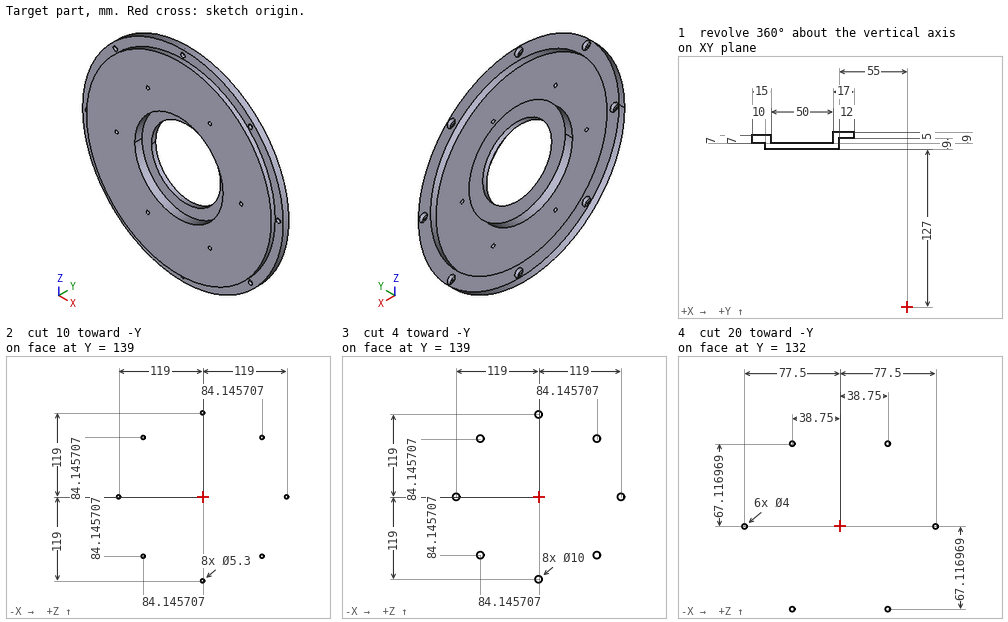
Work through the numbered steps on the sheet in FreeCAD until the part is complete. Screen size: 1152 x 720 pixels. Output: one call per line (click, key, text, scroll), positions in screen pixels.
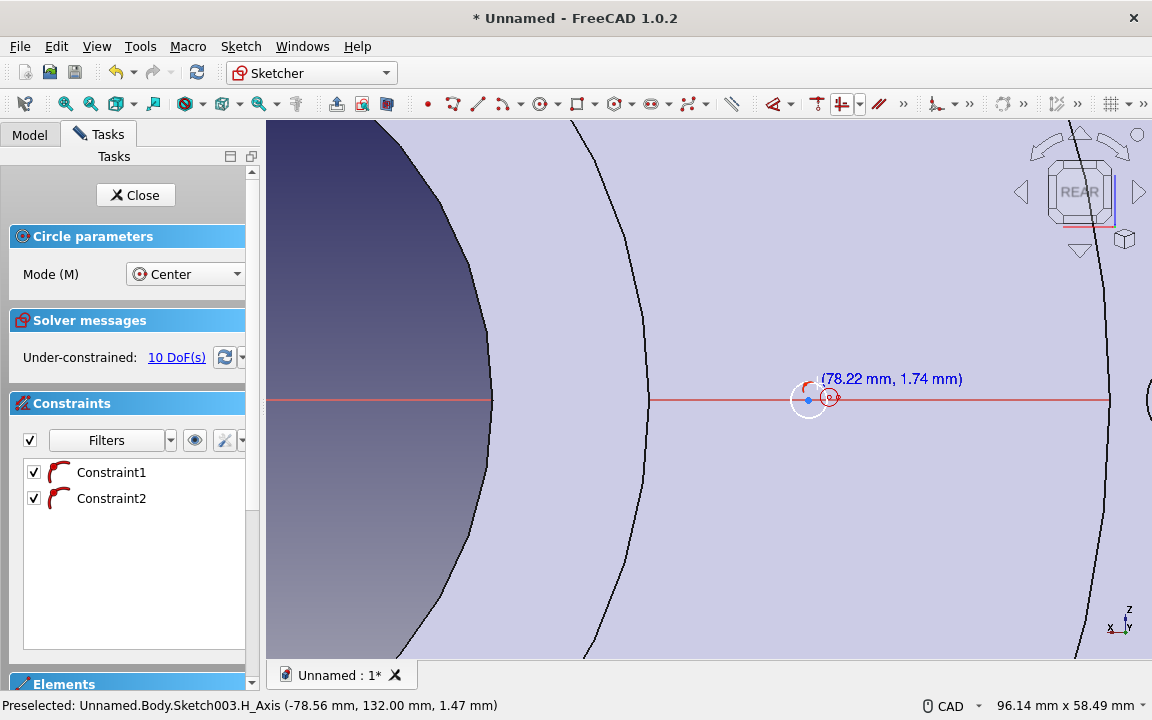
scroll(819, 386, down, 7)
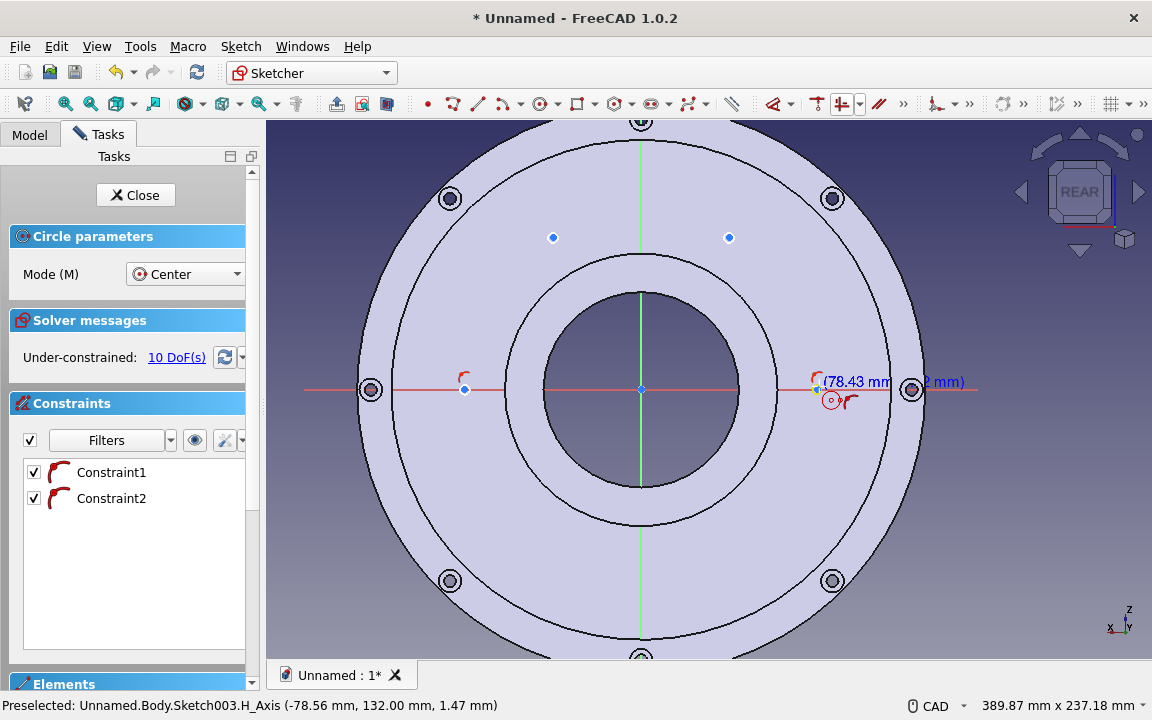
scroll(729, 542, up, 9)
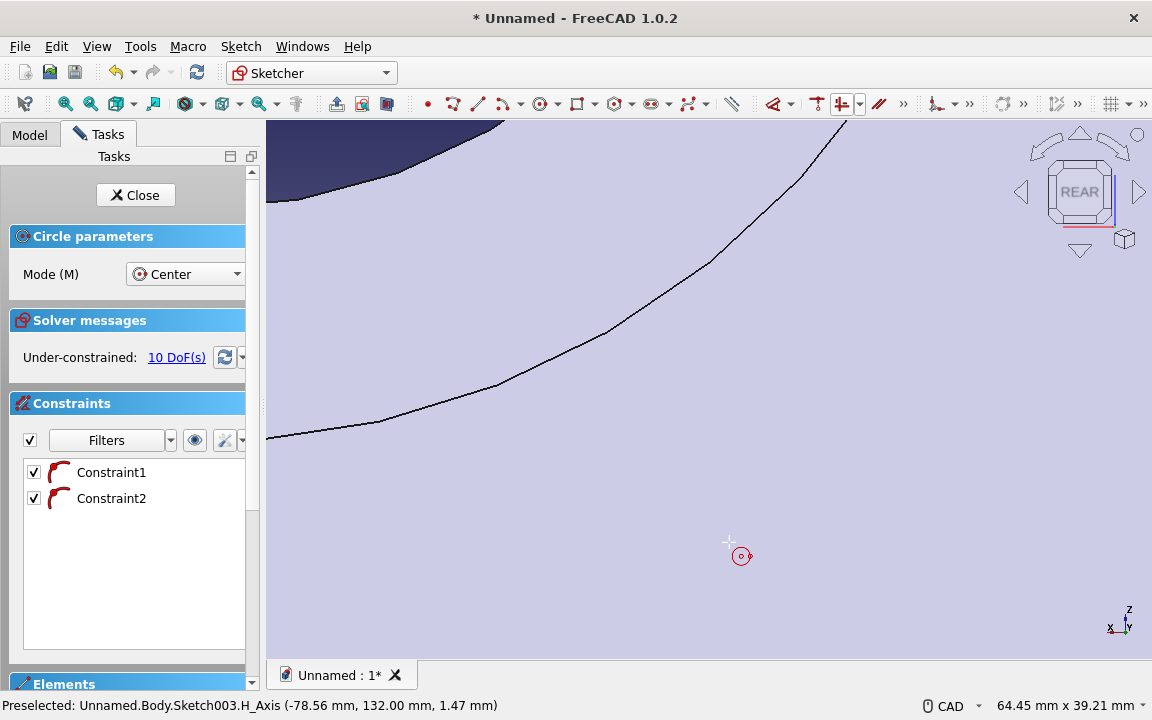
scroll(729, 542, down, 9)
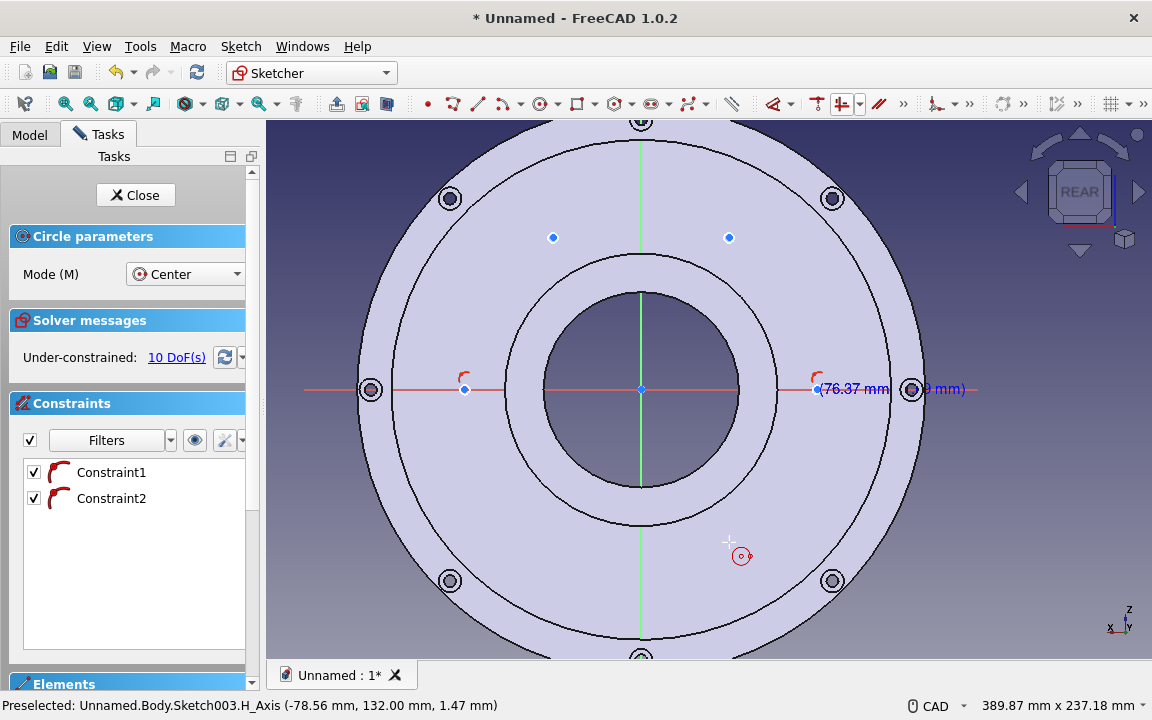
click(729, 542)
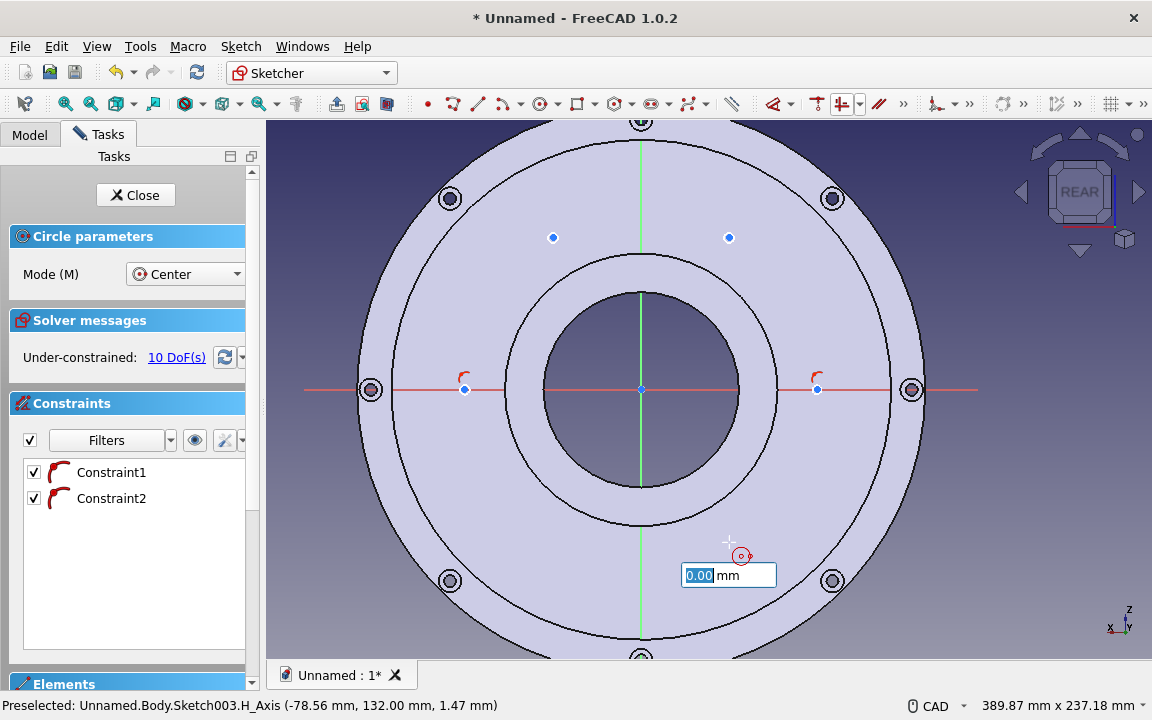
scroll(733, 539, up, 7)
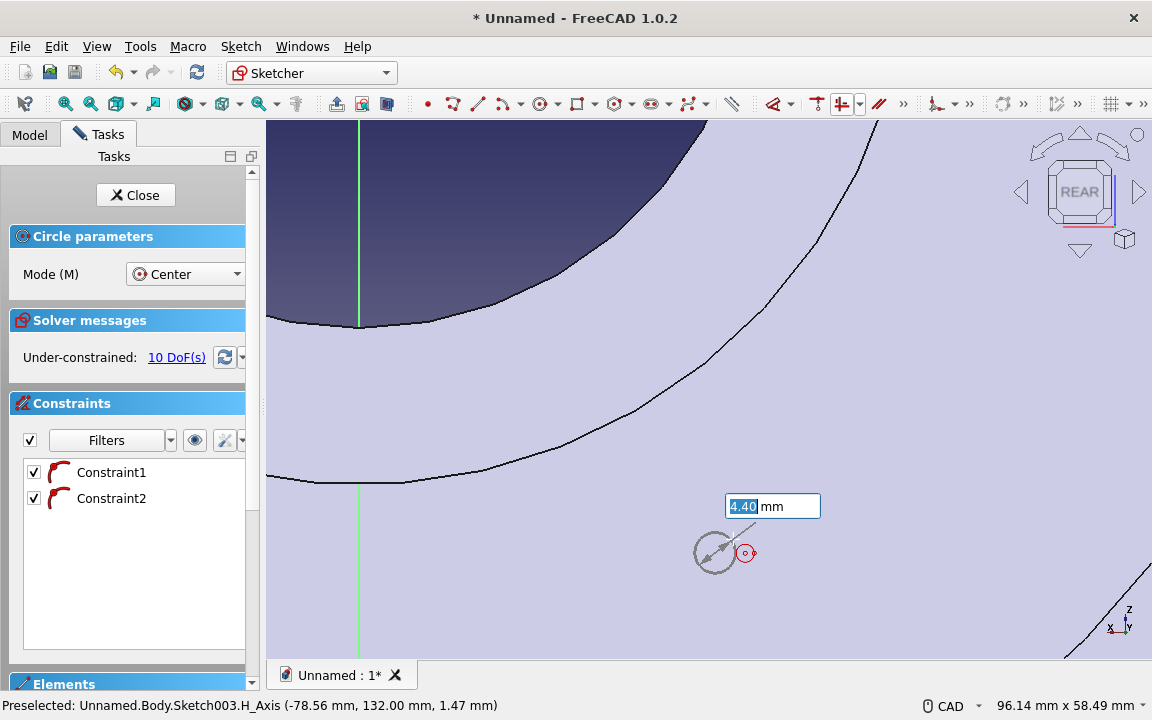
click(729, 537)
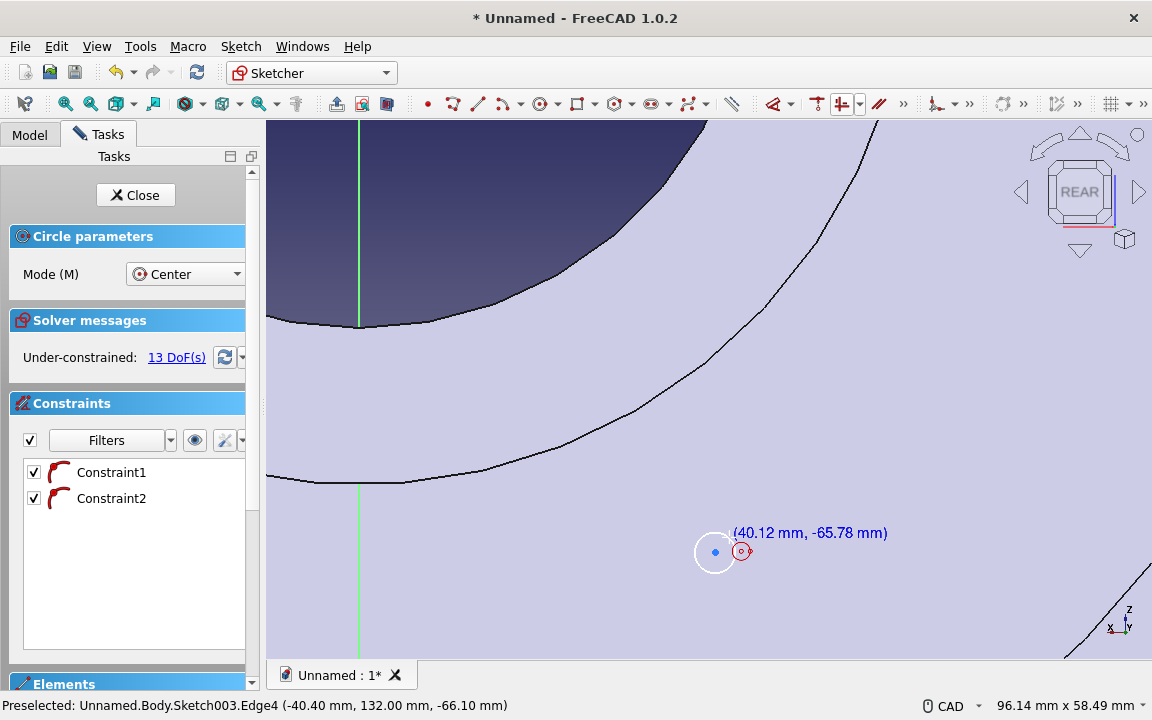
scroll(733, 539, down, 7)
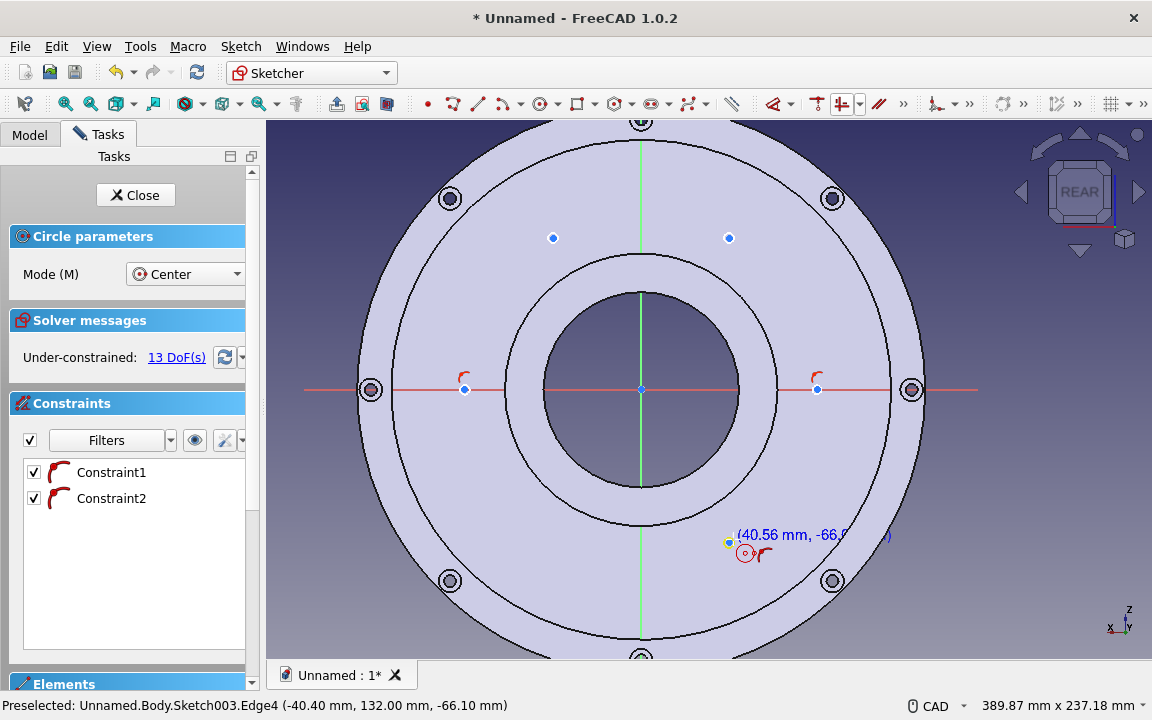
scroll(553, 542, up, 9)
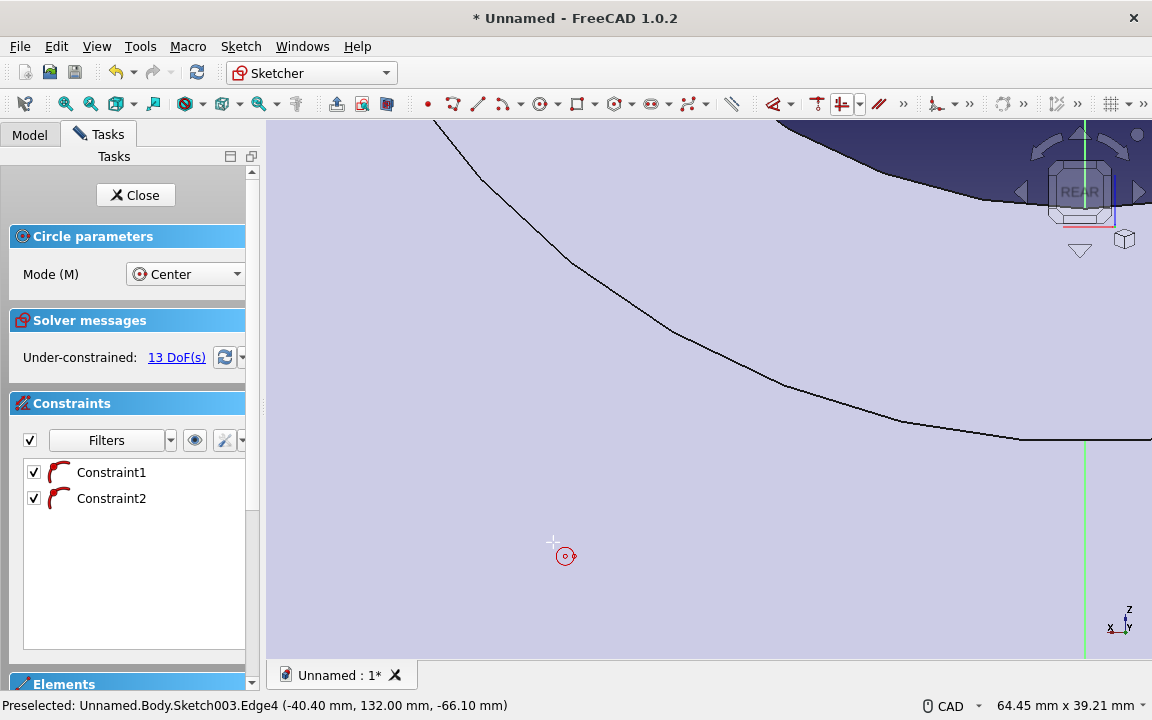
scroll(552, 542, down, 9)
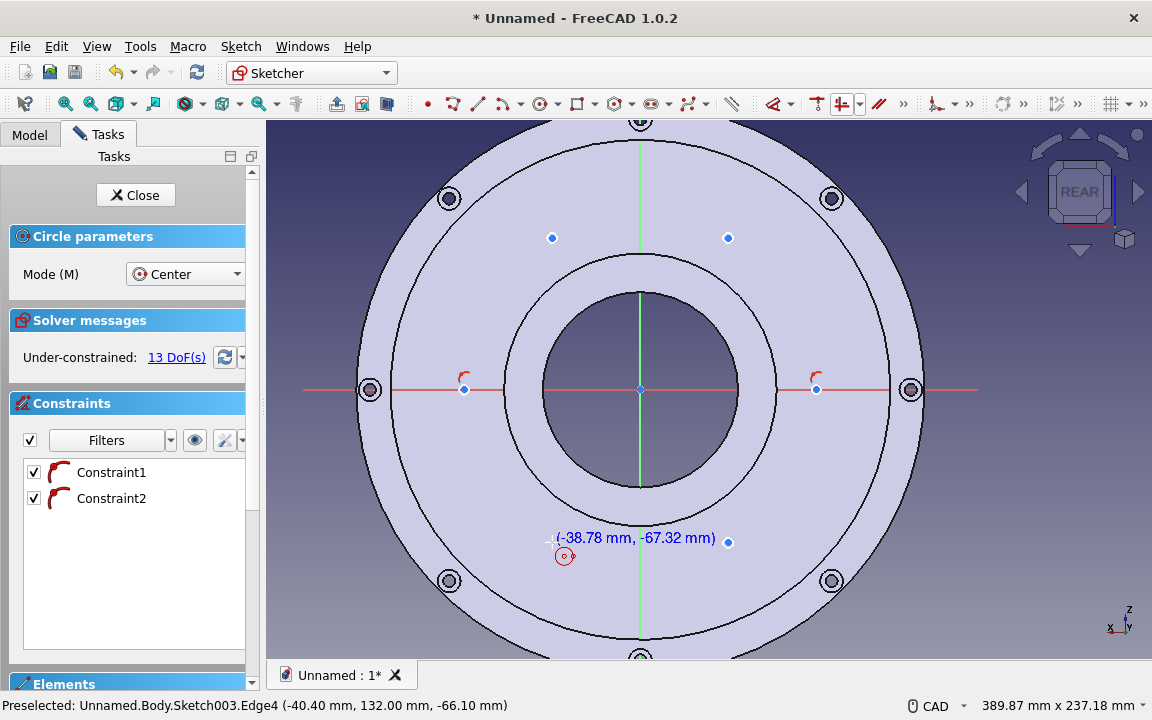
click(552, 542)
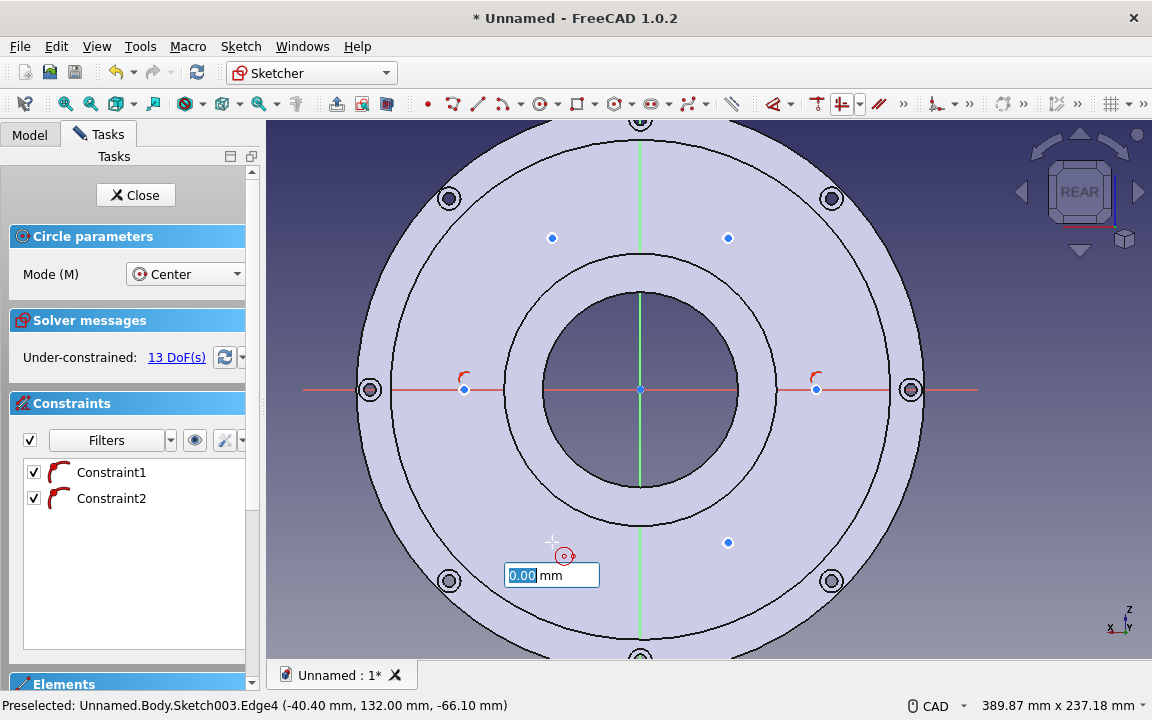
scroll(556, 539, up, 7)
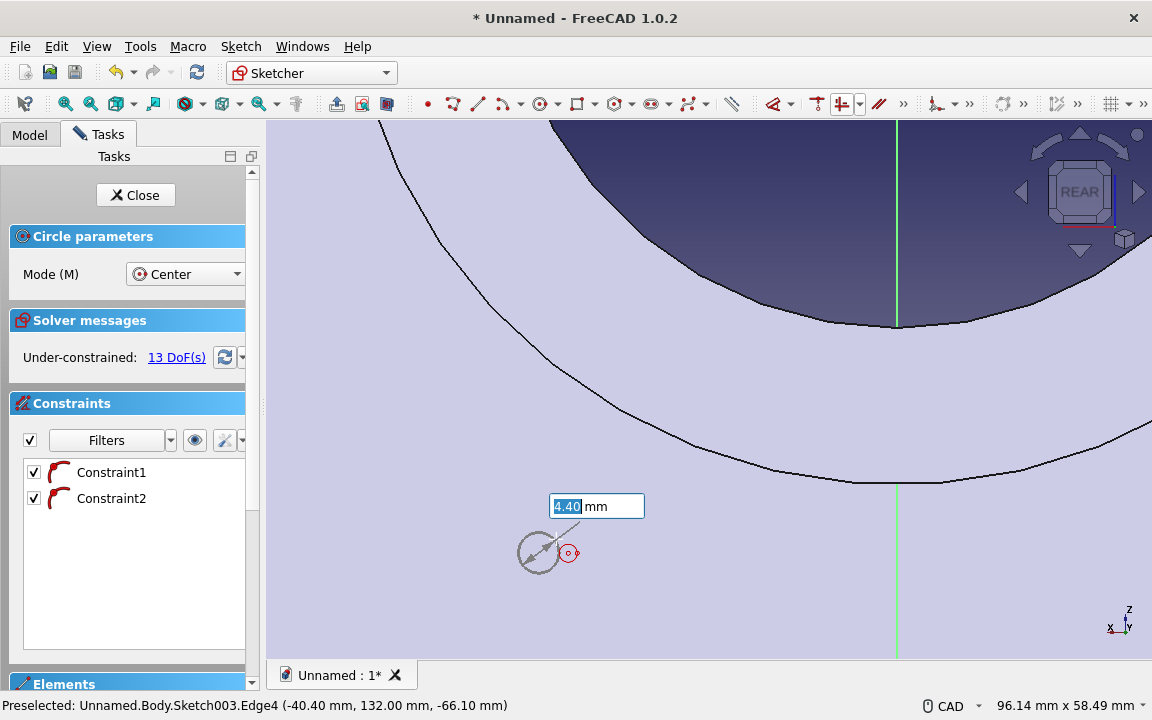
click(553, 537)
key(Escape)